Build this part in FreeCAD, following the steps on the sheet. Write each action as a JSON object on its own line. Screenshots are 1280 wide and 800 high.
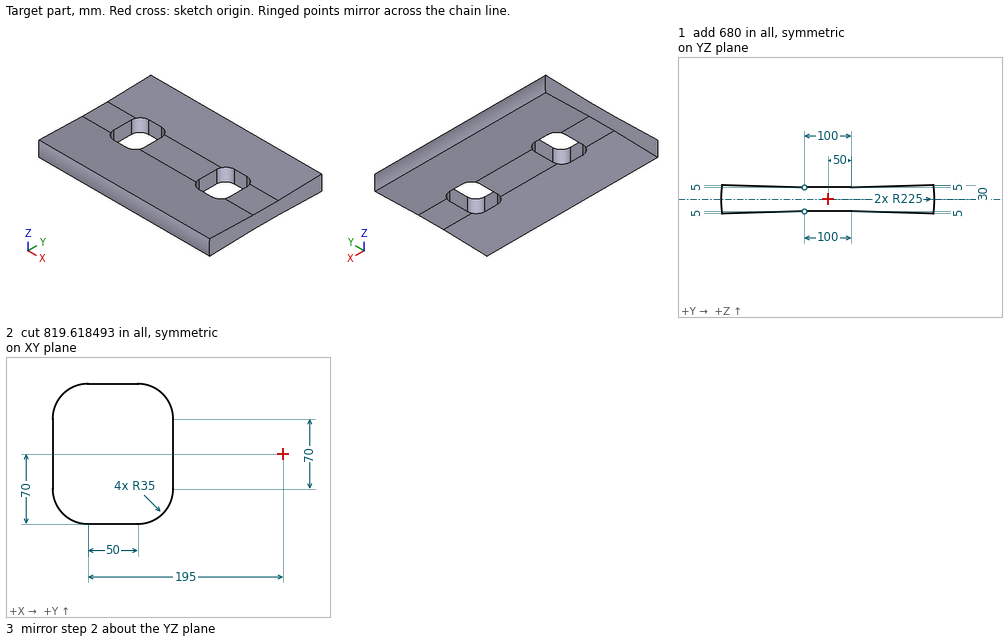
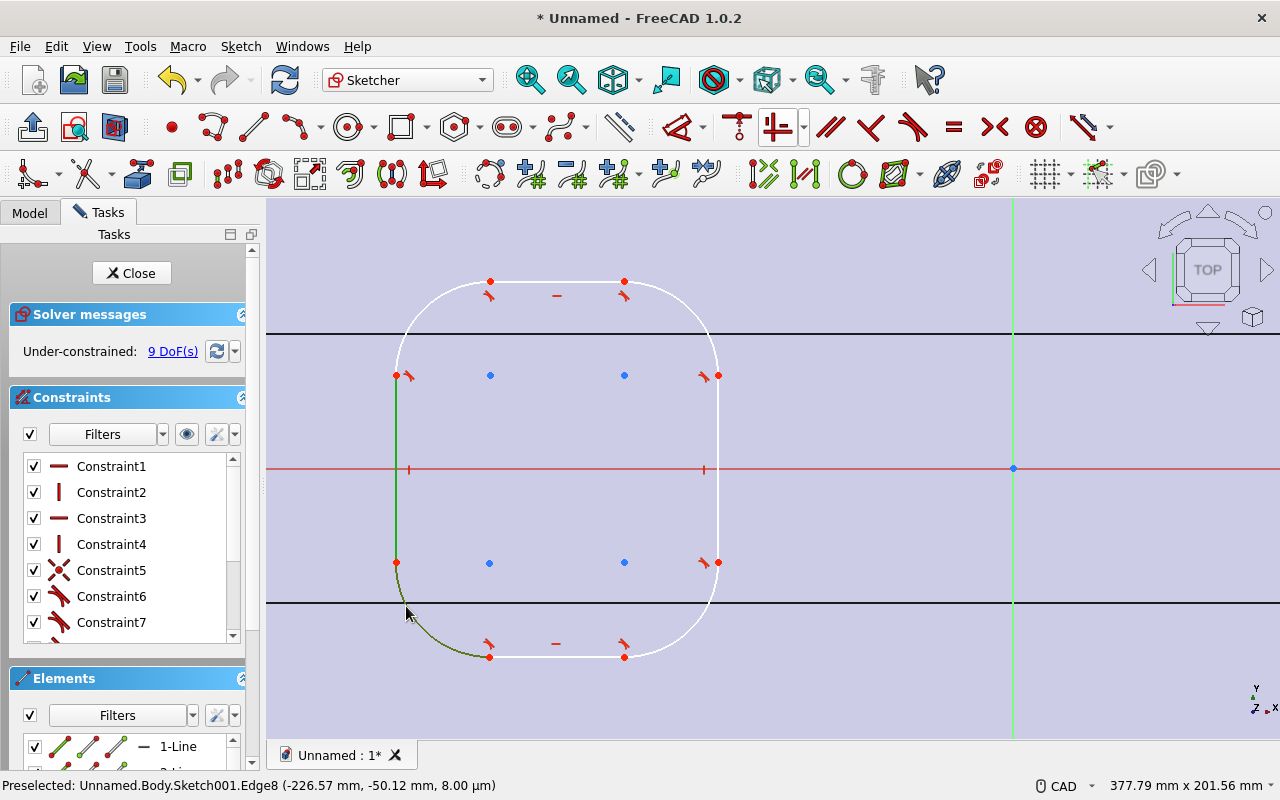
{"action": "left_click", "coordinate": [913, 128]}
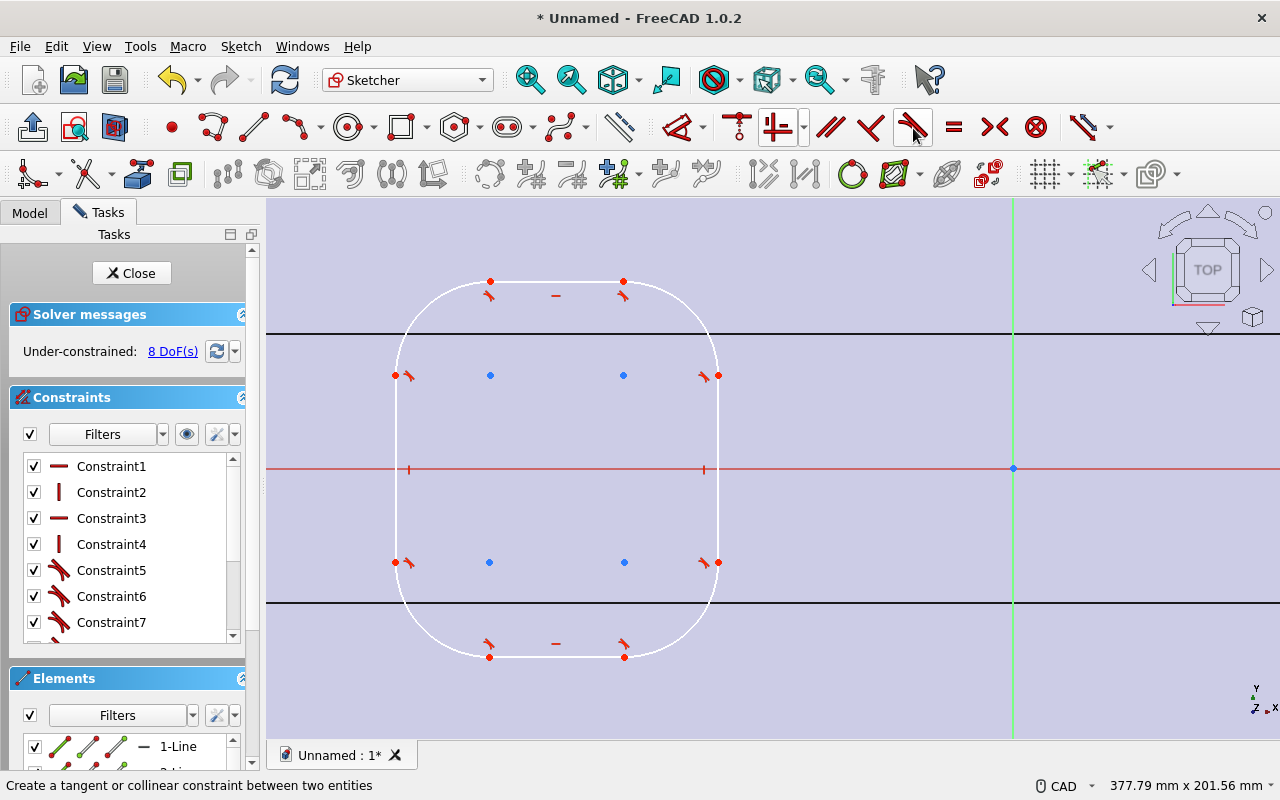
{"action": "left_click", "coordinate": [667, 647]}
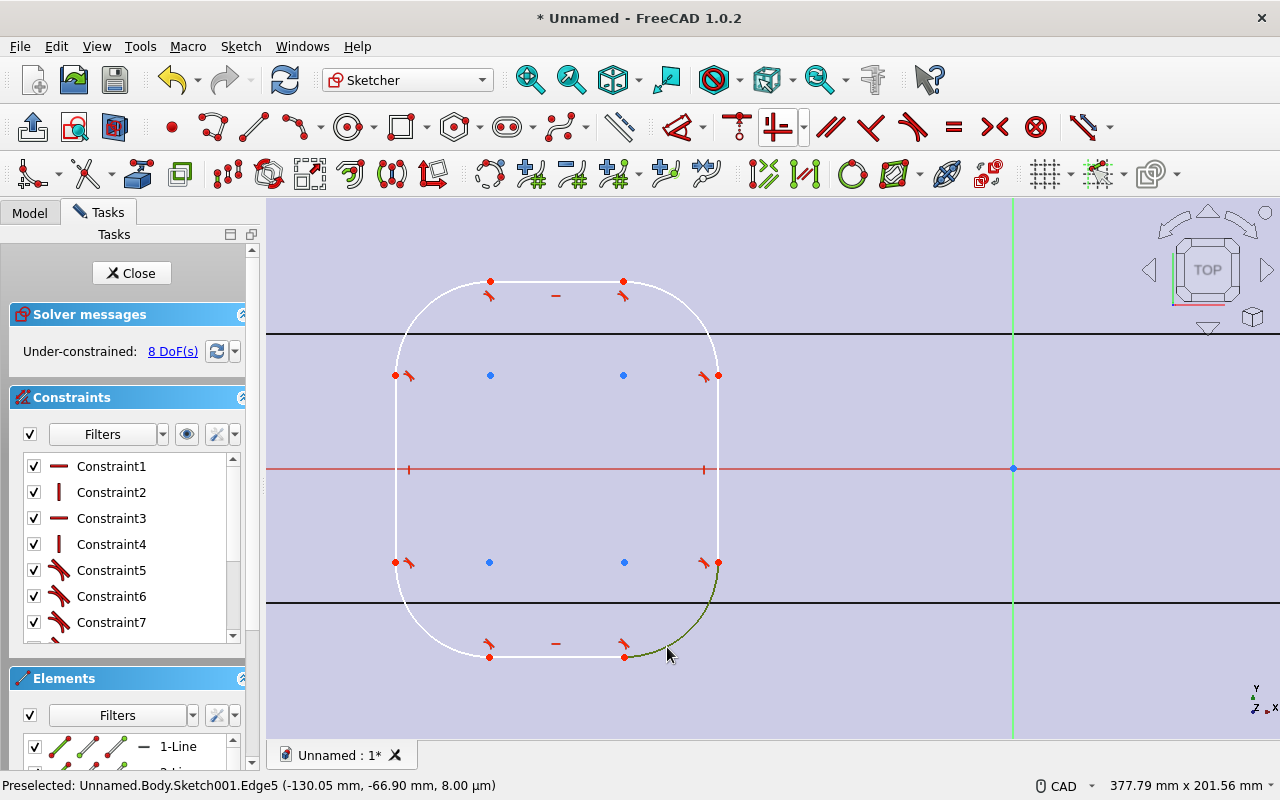
{"action": "left_click", "coordinate": [708, 333]}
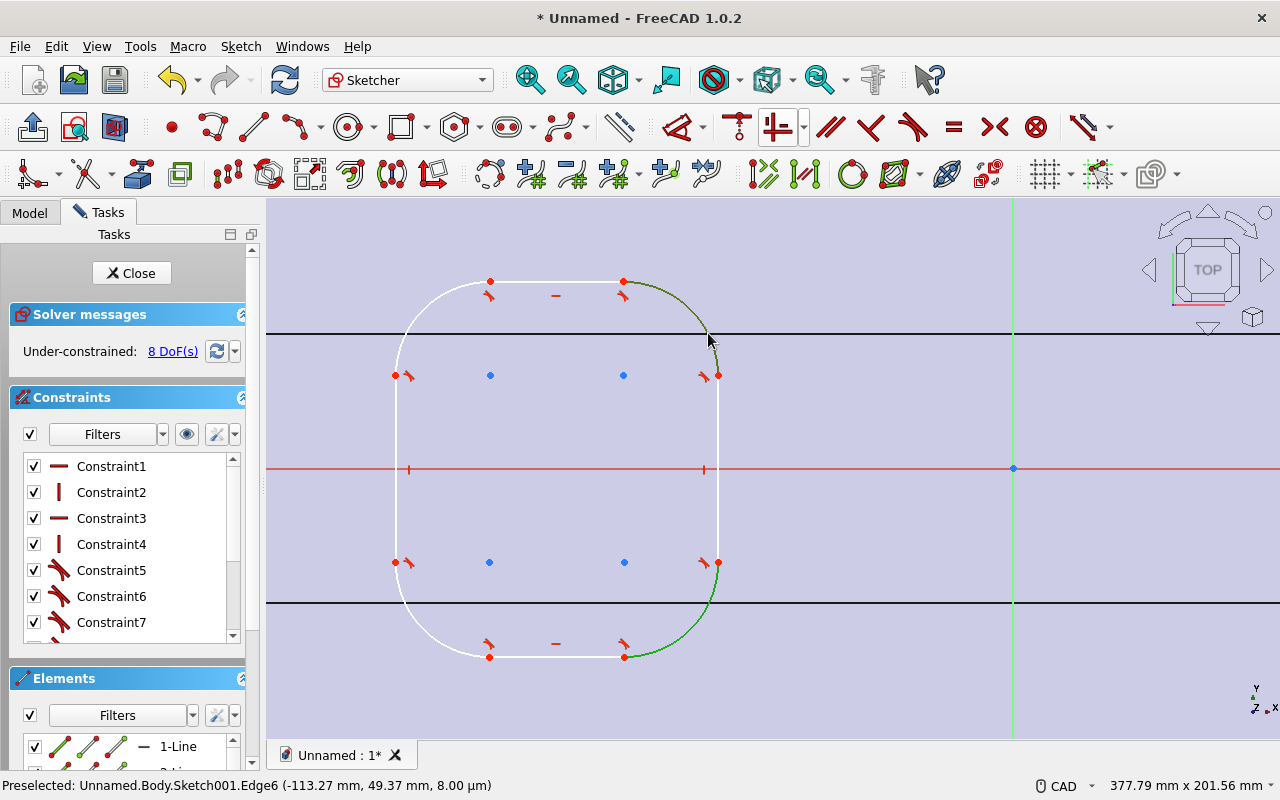
{"action": "left_click", "coordinate": [447, 292]}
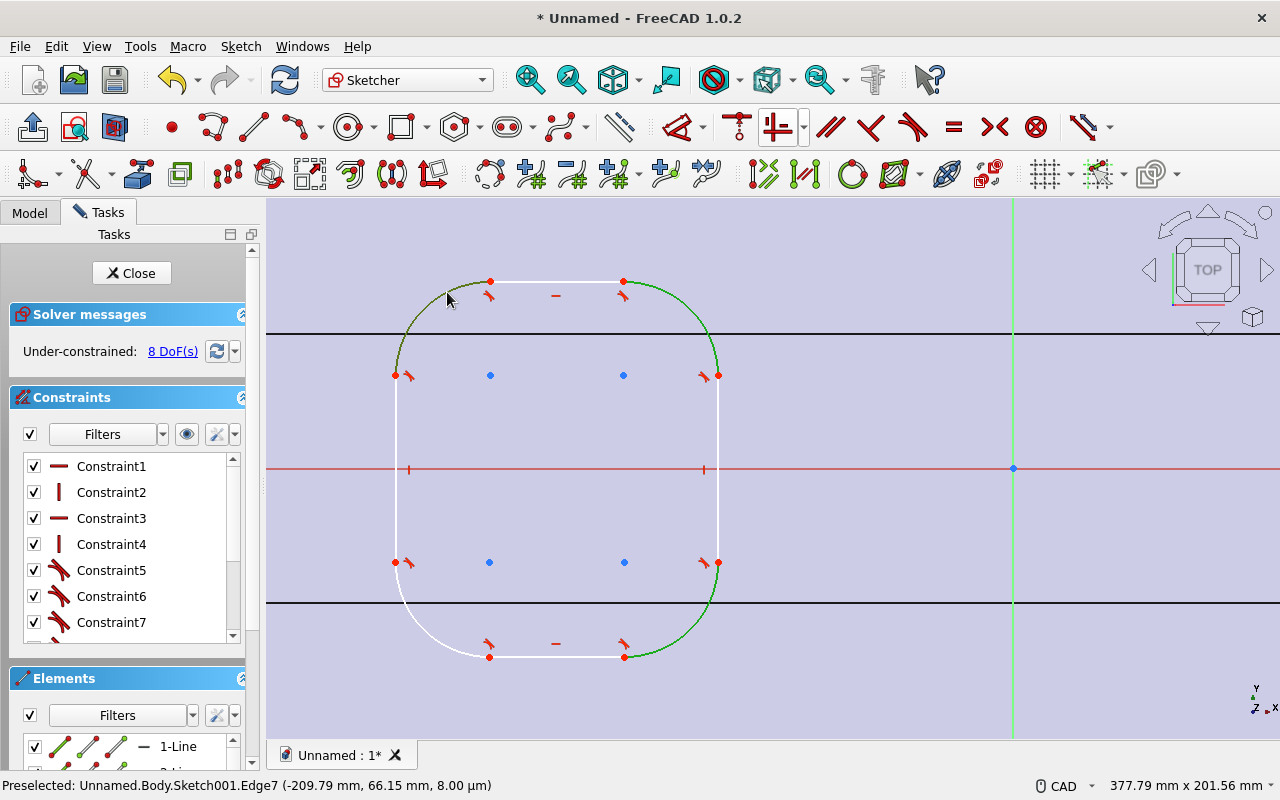
{"action": "left_click", "coordinate": [406, 606]}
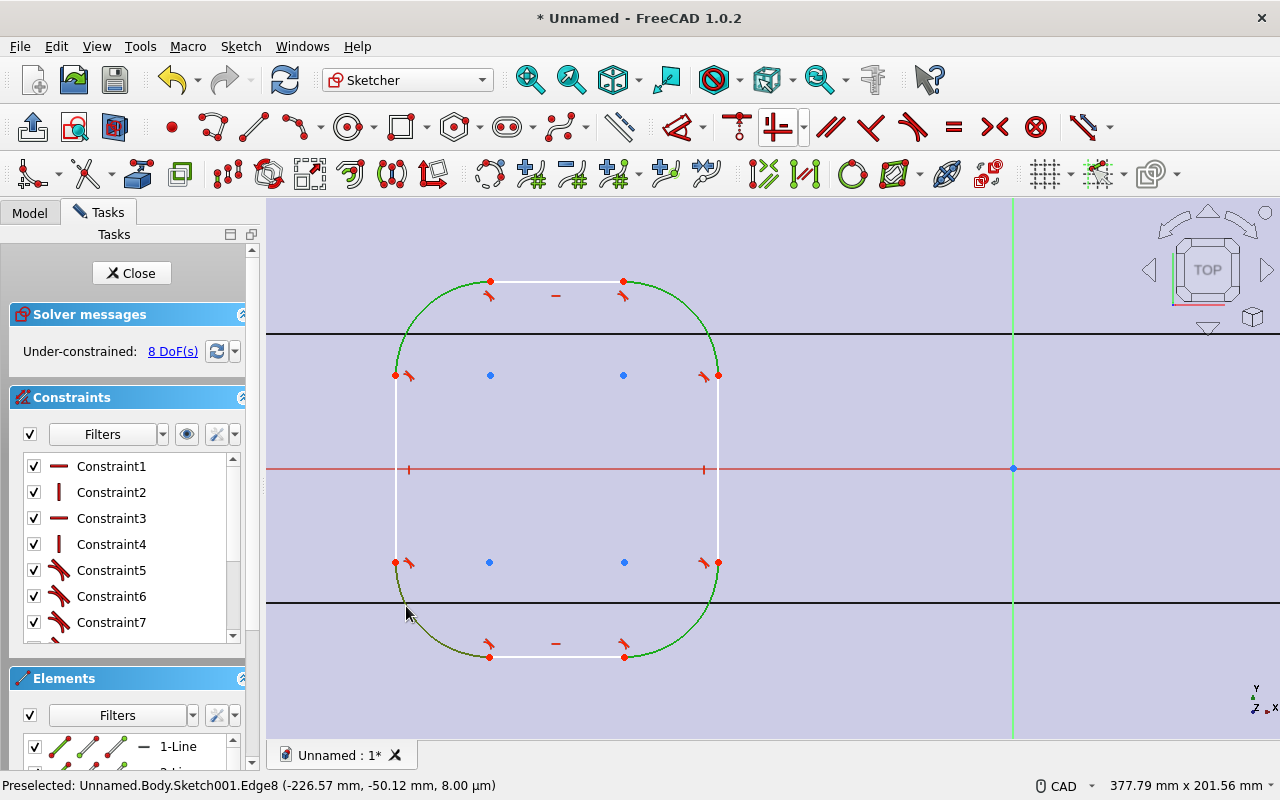
{"action": "key", "text": "e"}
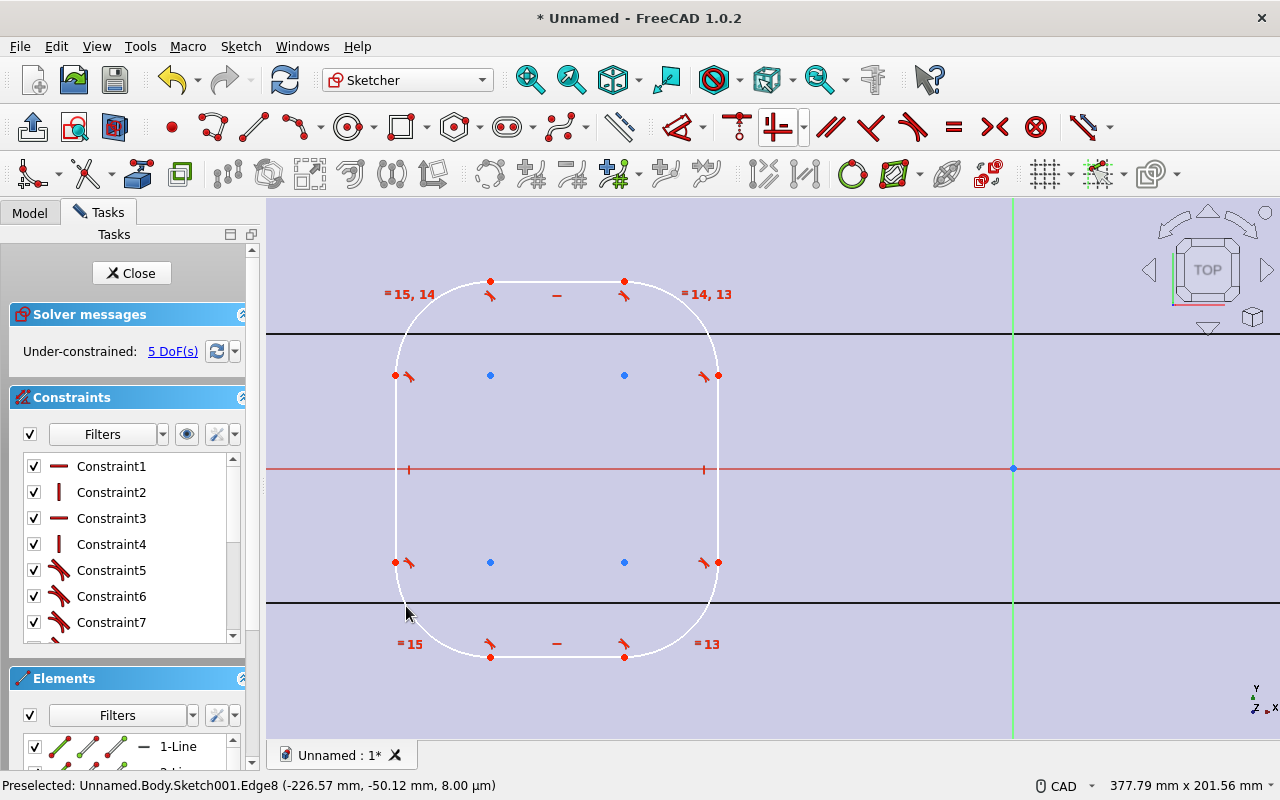
{"action": "left_click", "coordinate": [667, 647]}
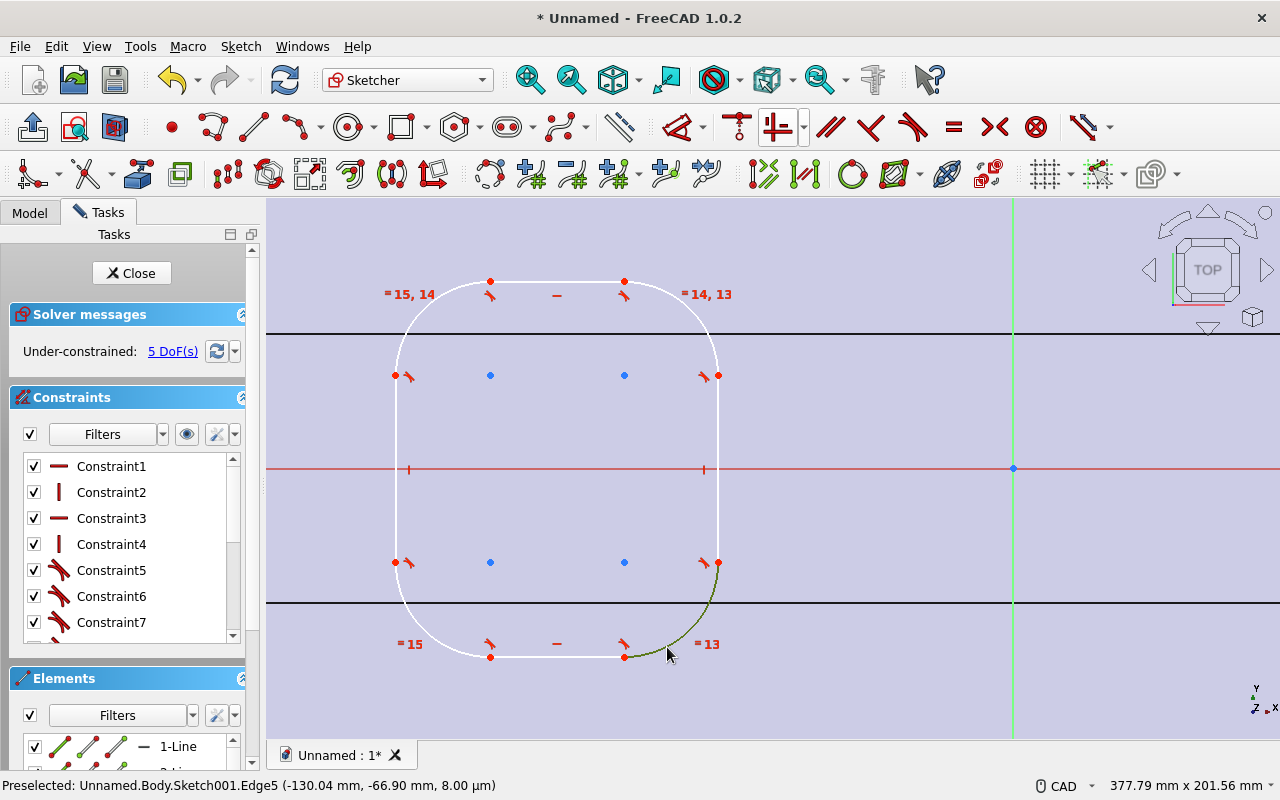
{"action": "key", "text": "k r"}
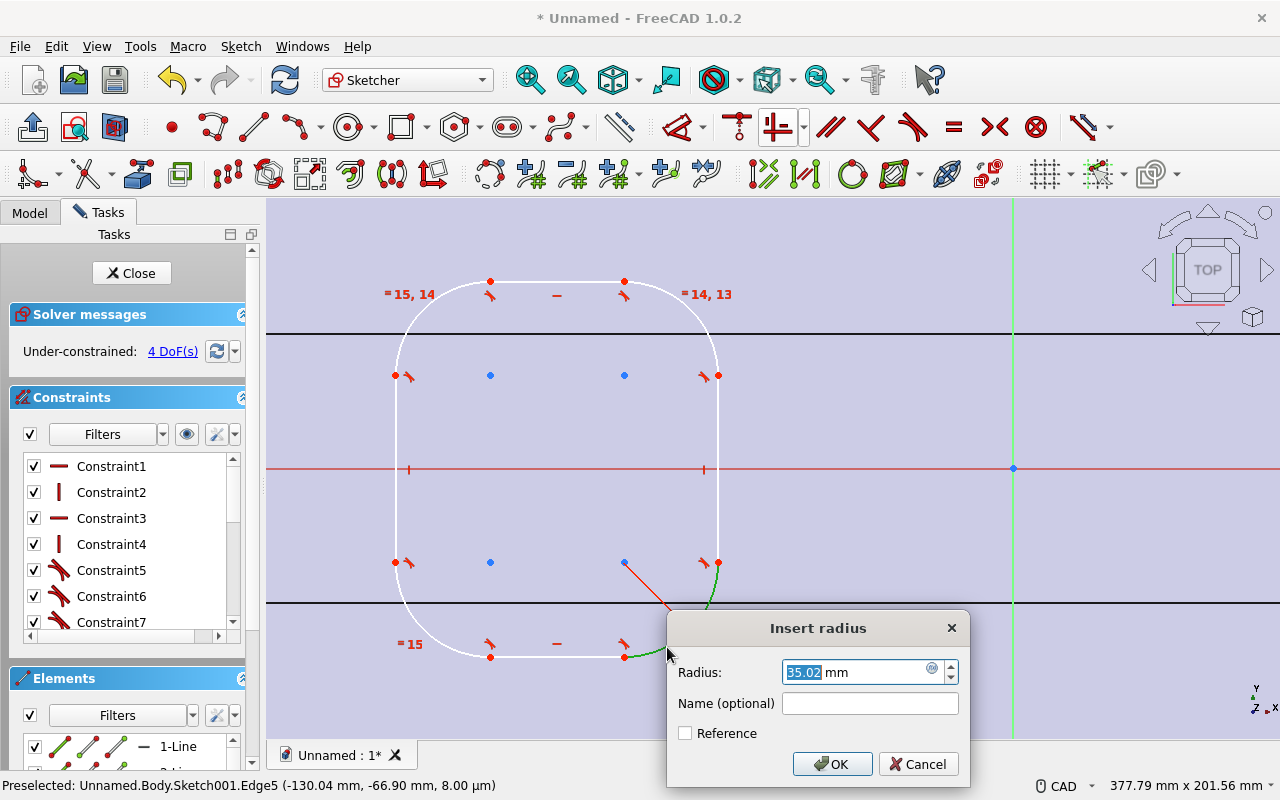
{"action": "type", "text": "35"}
{"action": "key", "text": "Return"}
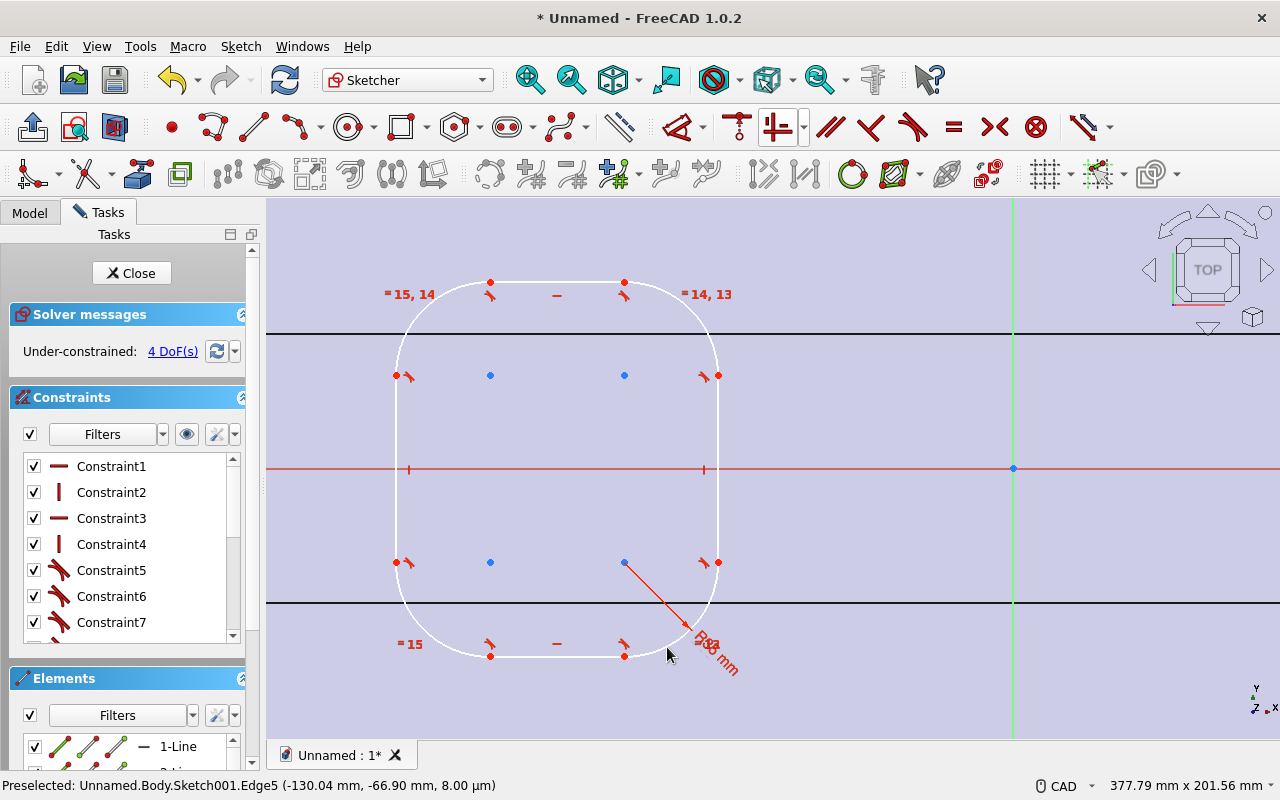
{"action": "left_click", "coordinate": [530, 657]}